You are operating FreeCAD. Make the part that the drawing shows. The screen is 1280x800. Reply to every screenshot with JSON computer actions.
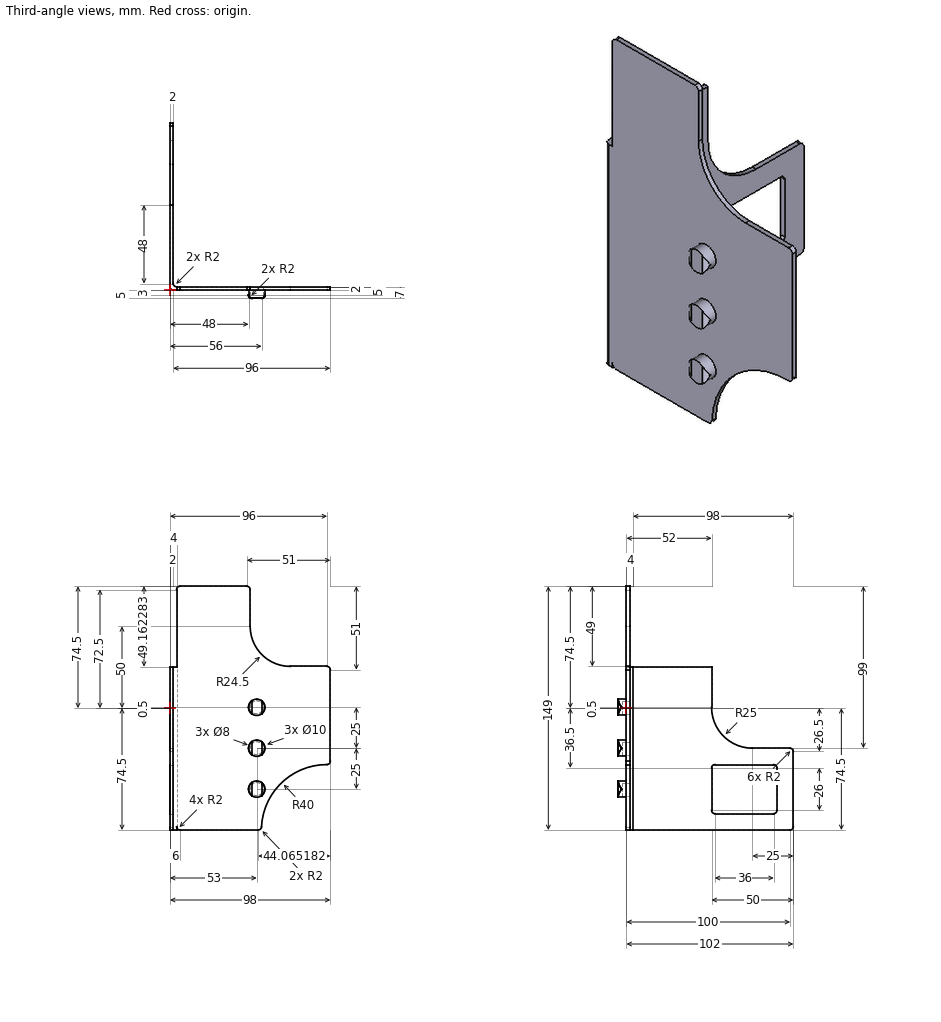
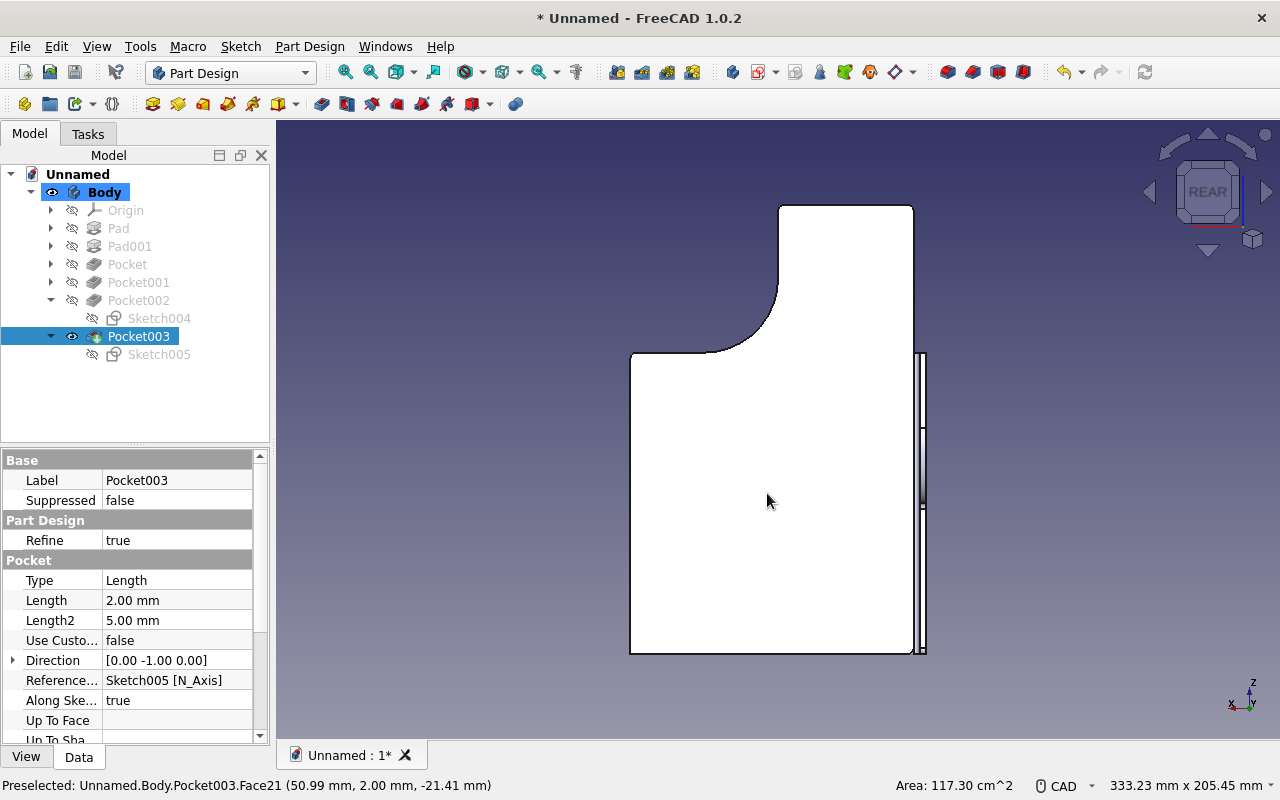
{"action": "left_click", "coordinate": [758, 72]}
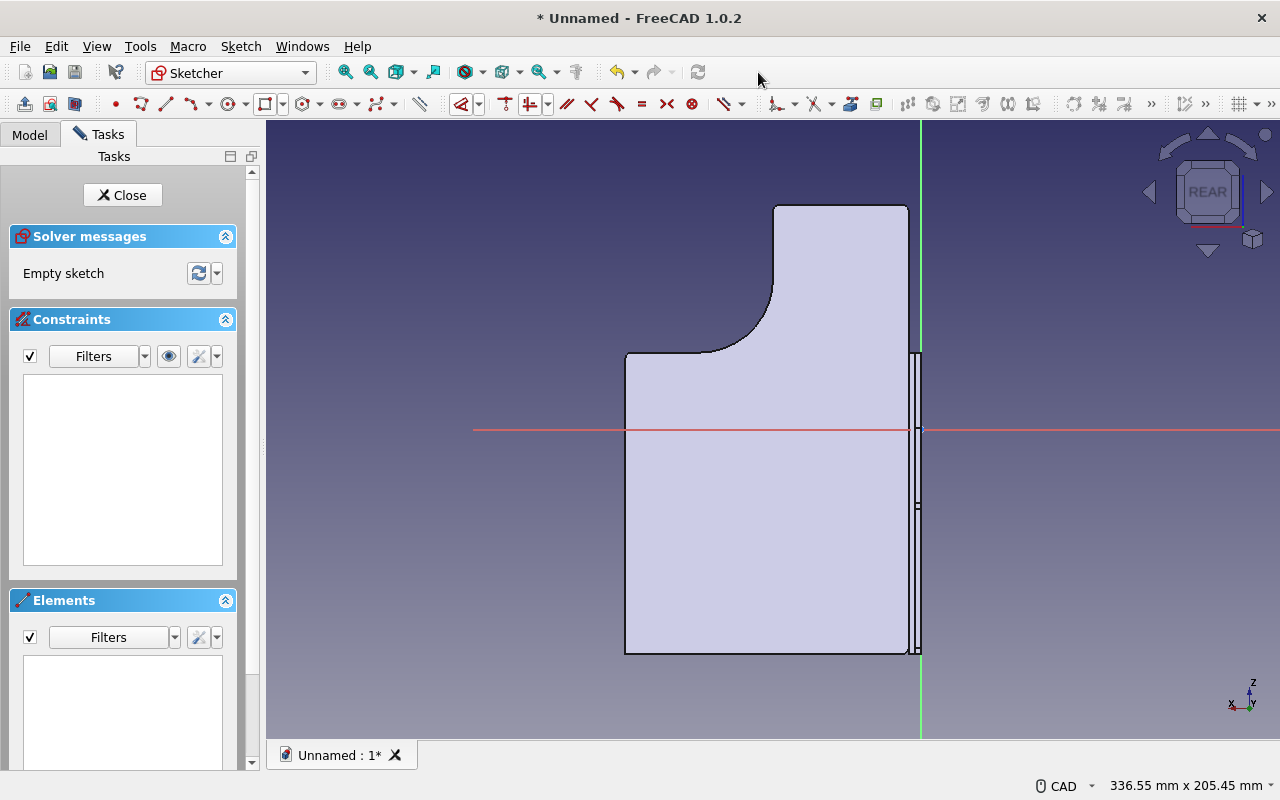
{"action": "scroll", "coordinate": [938, 564], "scroll_direction": "up", "scroll_amount": 4}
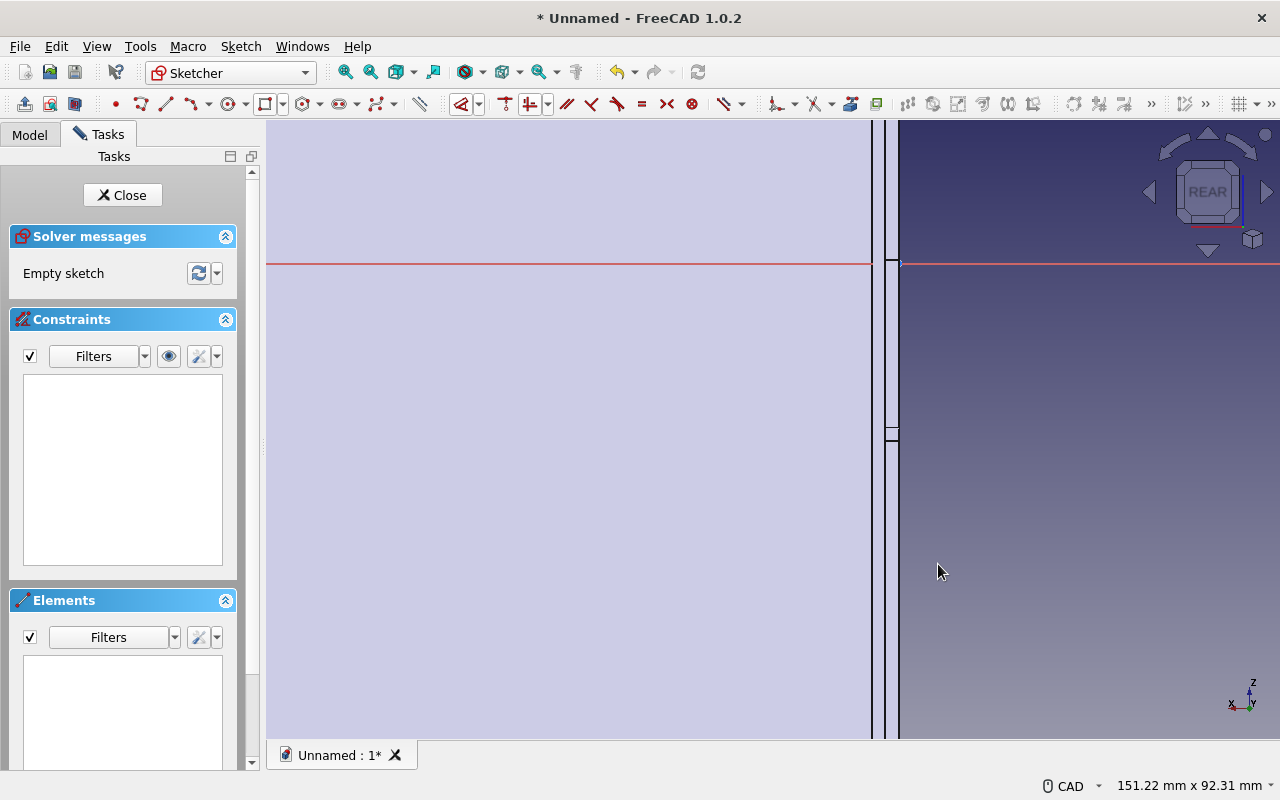
{"action": "key", "text": "g c"}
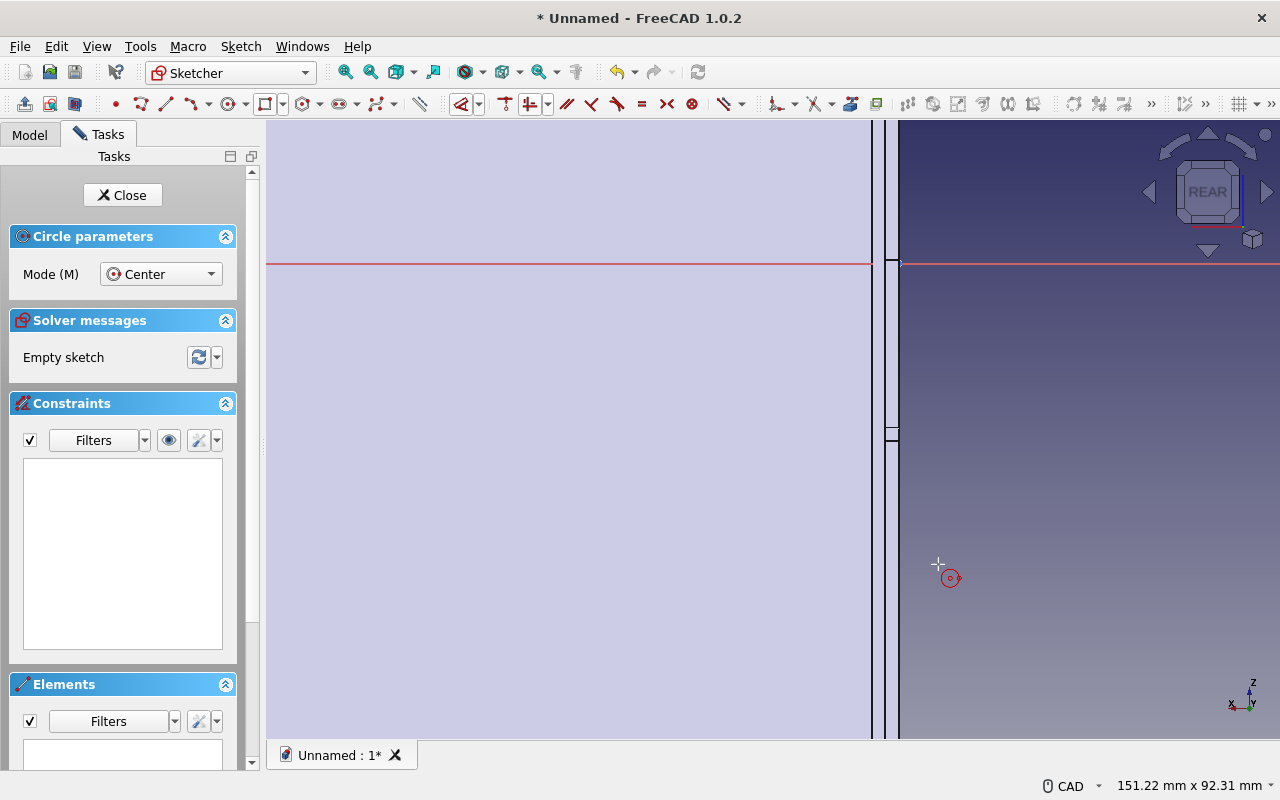
{"action": "left_click", "coordinate": [543, 428]}
{"action": "mouse_move", "coordinate": [567, 404]}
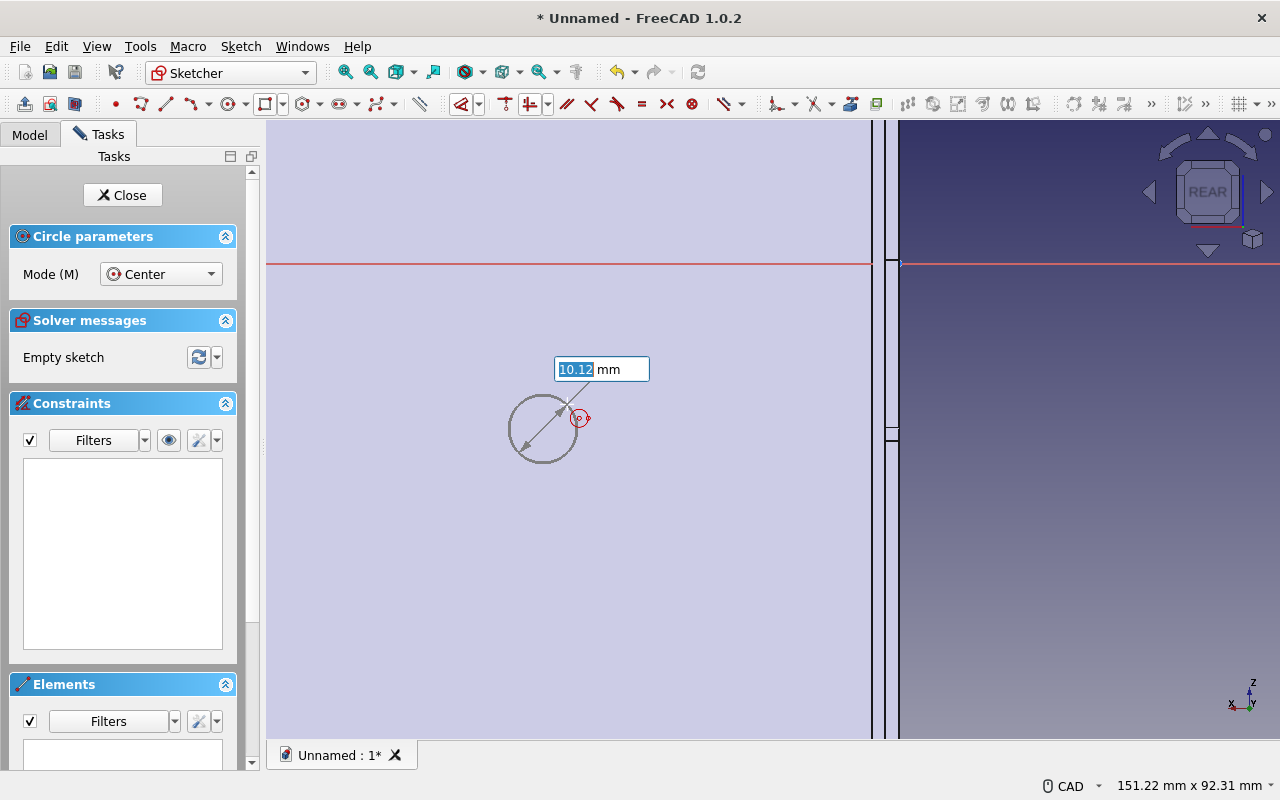
{"action": "type", "text": "10"}
{"action": "key", "text": "Return"}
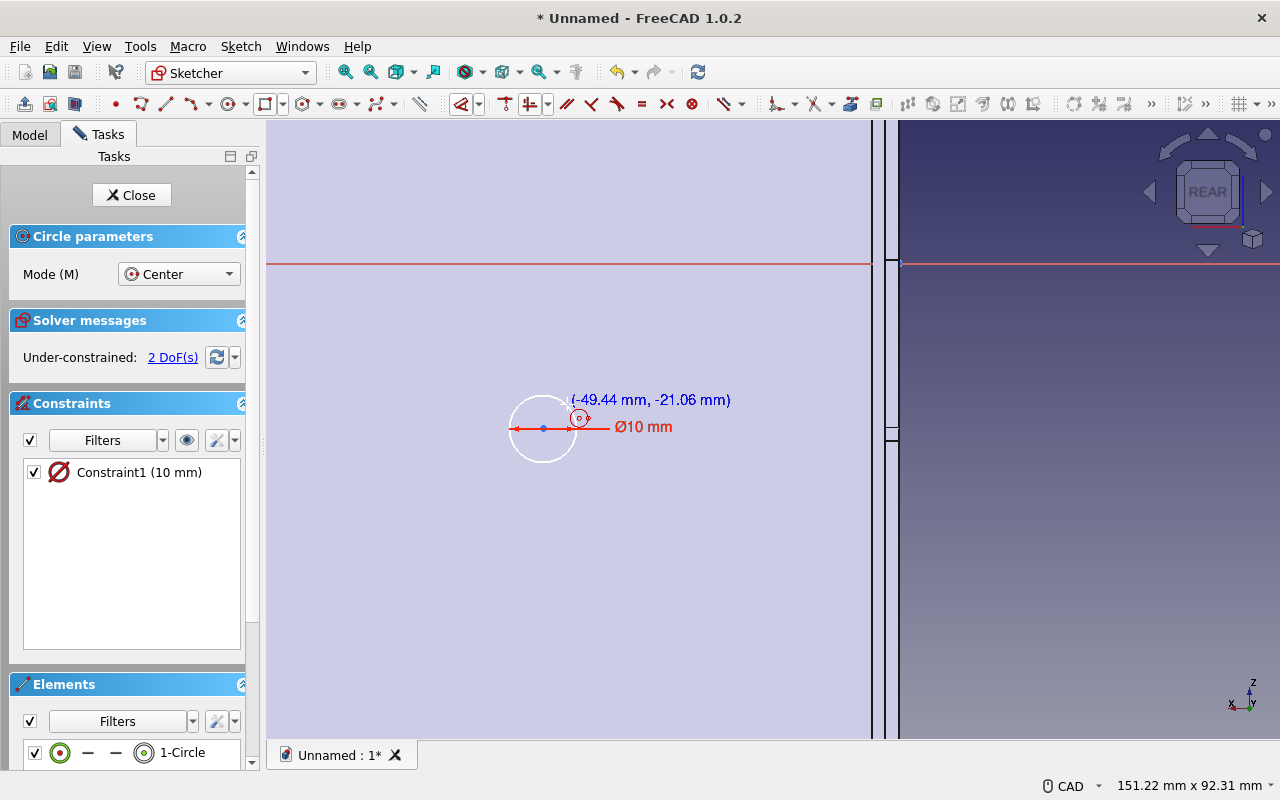
{"action": "left_click", "coordinate": [543, 596]}
{"action": "mouse_move", "coordinate": [567, 572]}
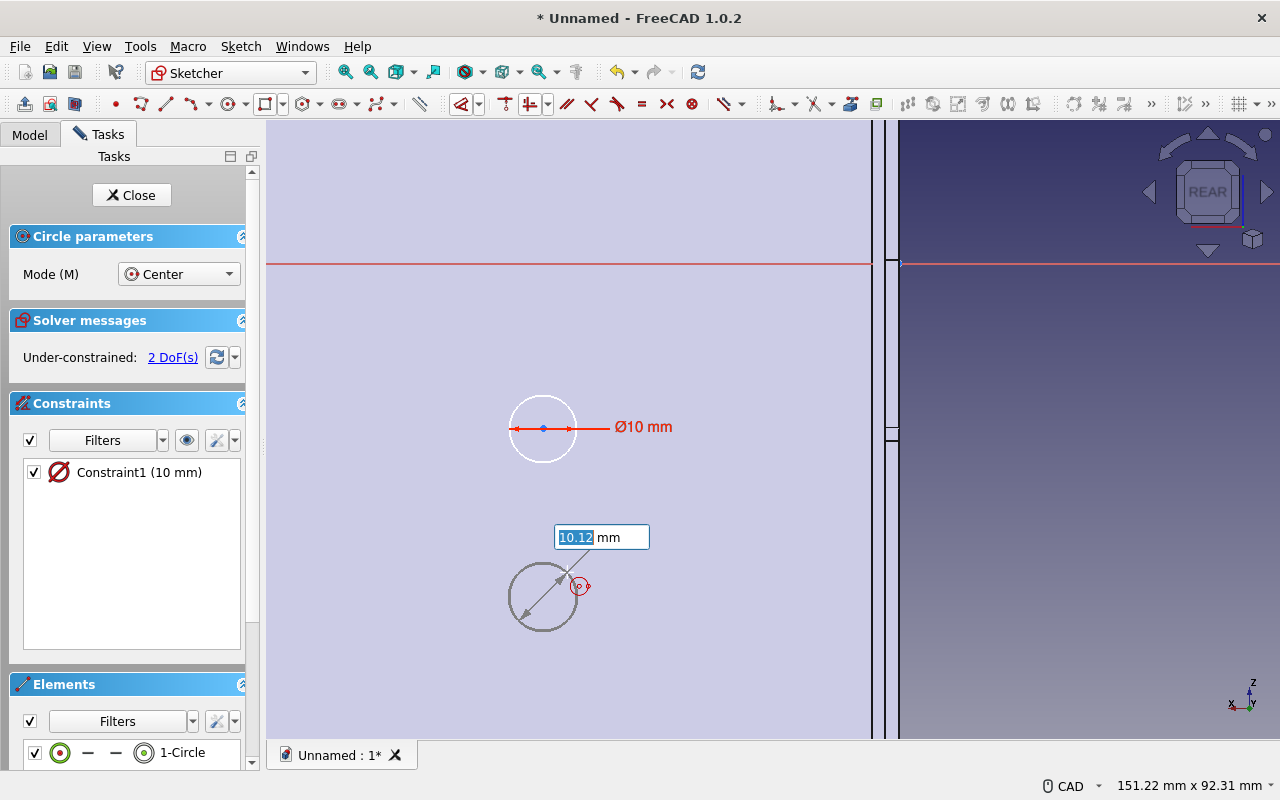
{"action": "type", "text": "10"}
{"action": "key", "text": "Return"}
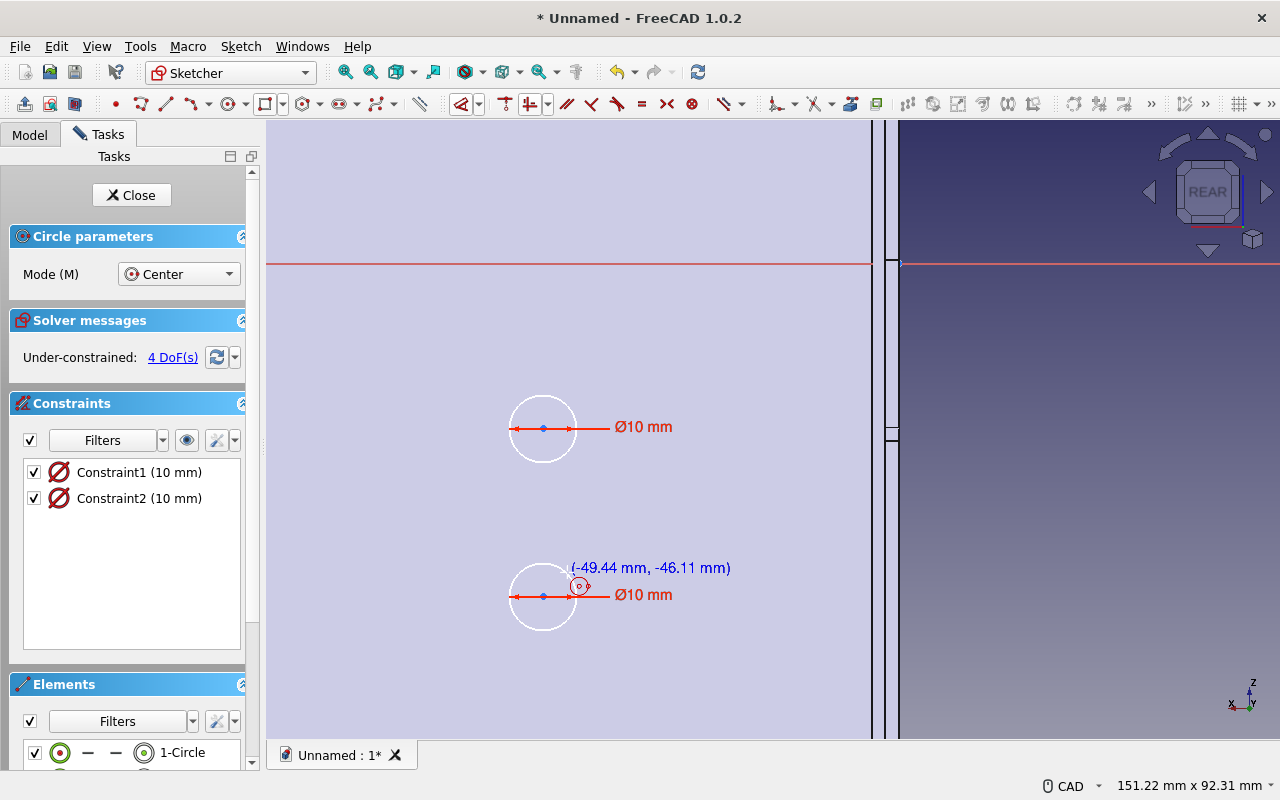
{"action": "scroll", "coordinate": [543, 260], "scroll_direction": "up", "scroll_amount": 8}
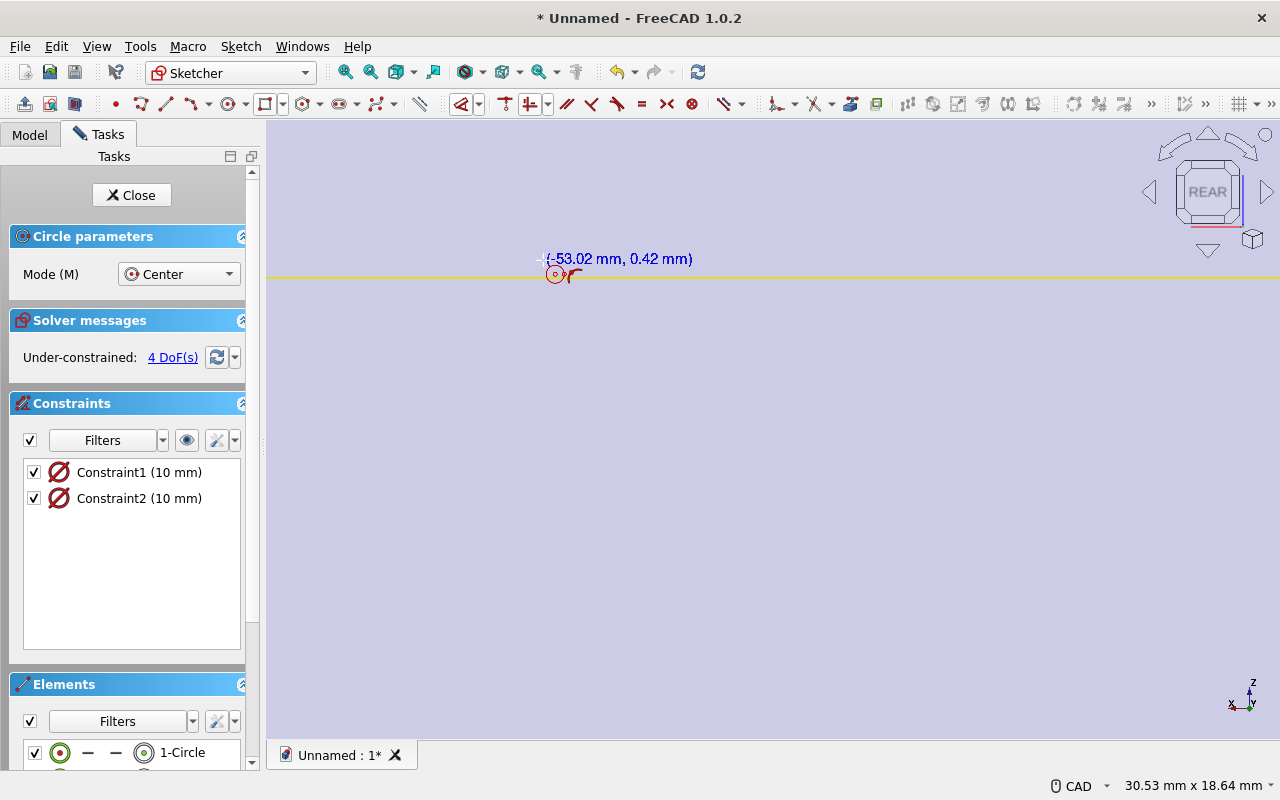
{"action": "left_click", "coordinate": [543, 261]}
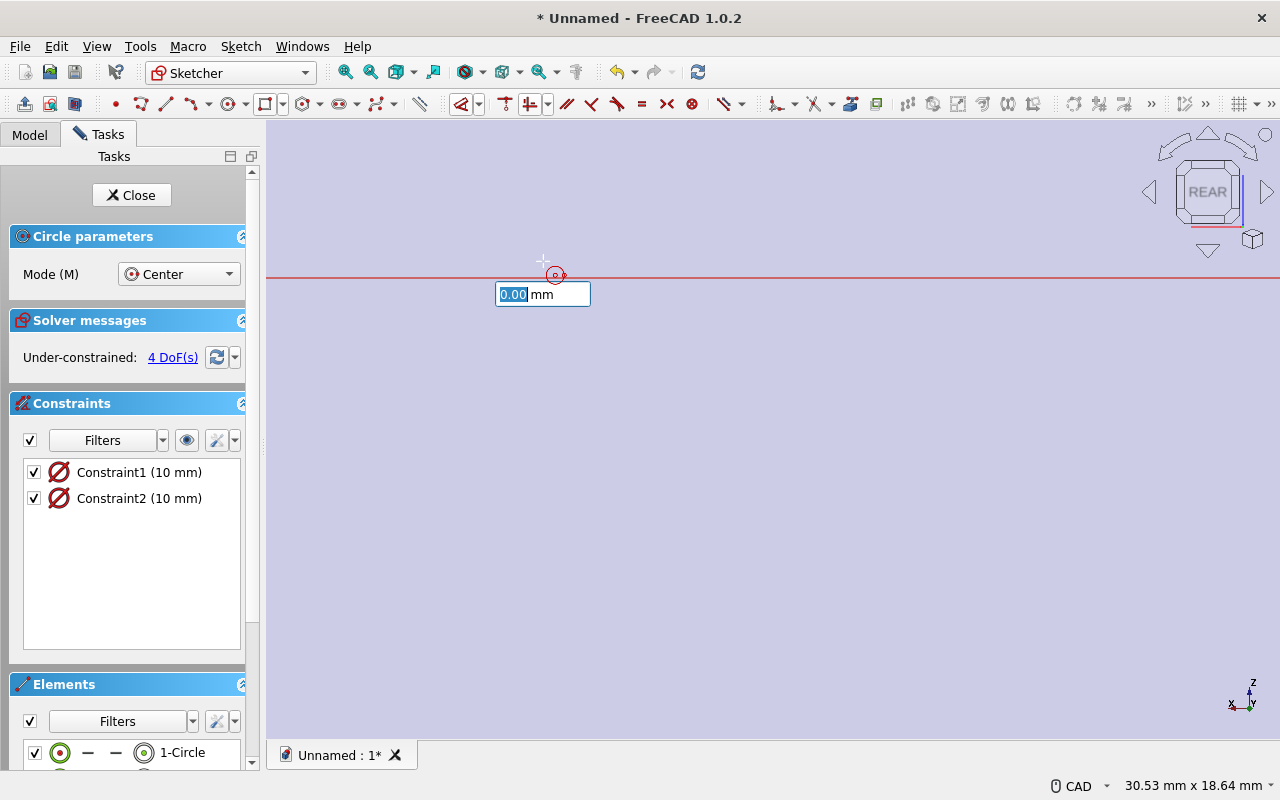
{"action": "scroll", "coordinate": [544, 262], "scroll_direction": "down", "scroll_amount": 8}
{"action": "mouse_move", "coordinate": [568, 238]}